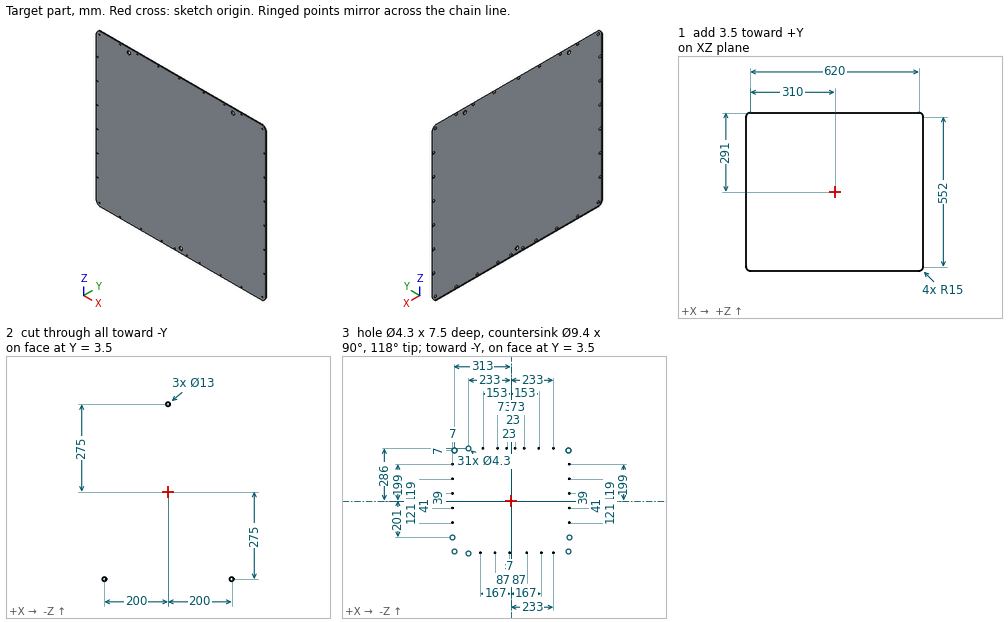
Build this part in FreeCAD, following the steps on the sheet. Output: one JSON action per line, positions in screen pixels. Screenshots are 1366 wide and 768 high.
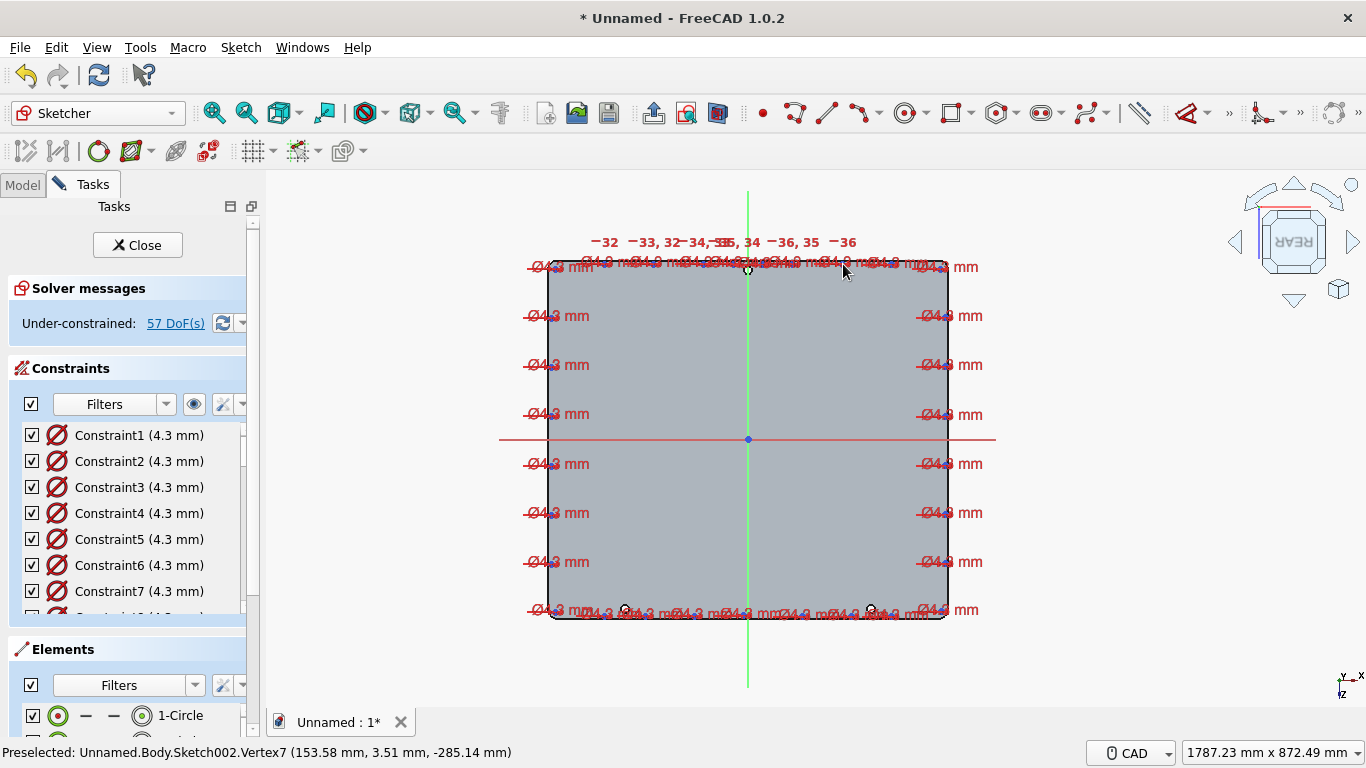
{"action": "left_click", "coordinate": [552, 318]}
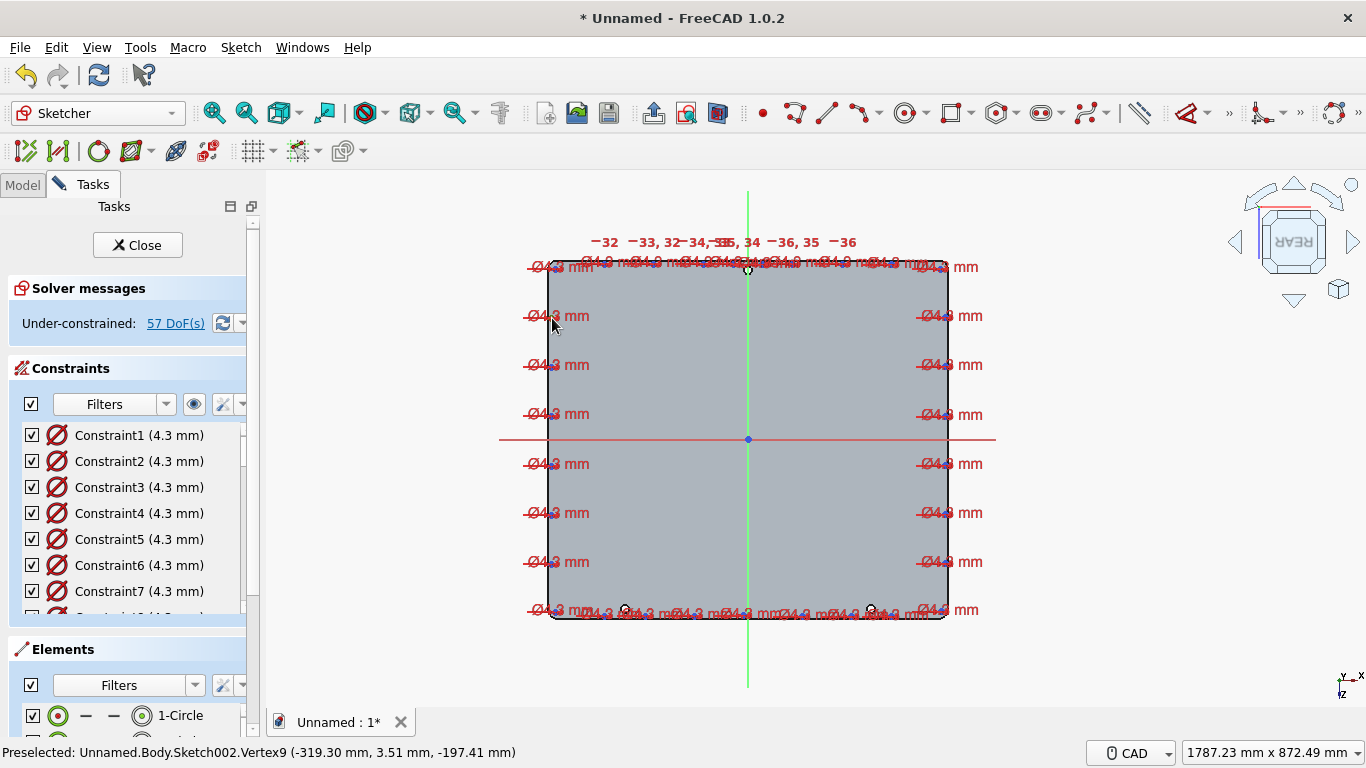
{"action": "left_click", "coordinate": [552, 367]}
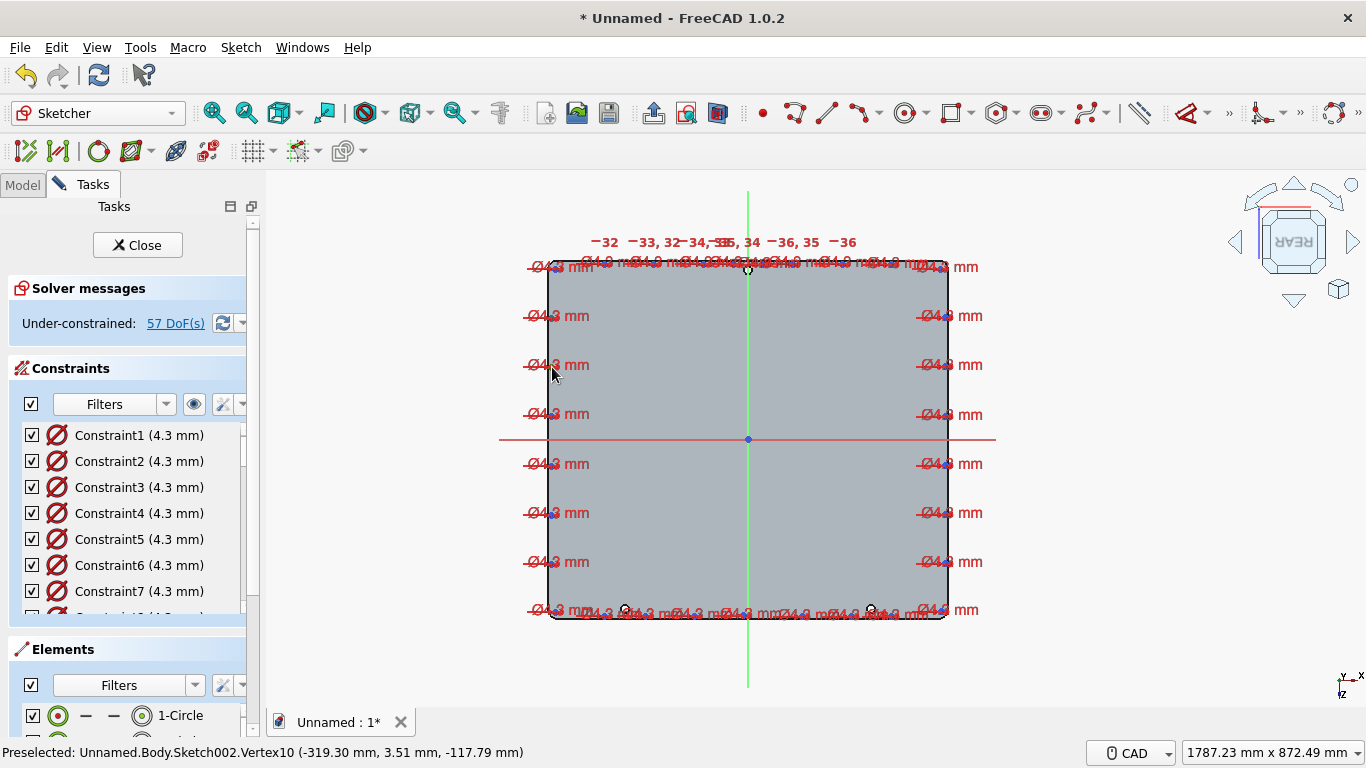
{"action": "key", "text": "v"}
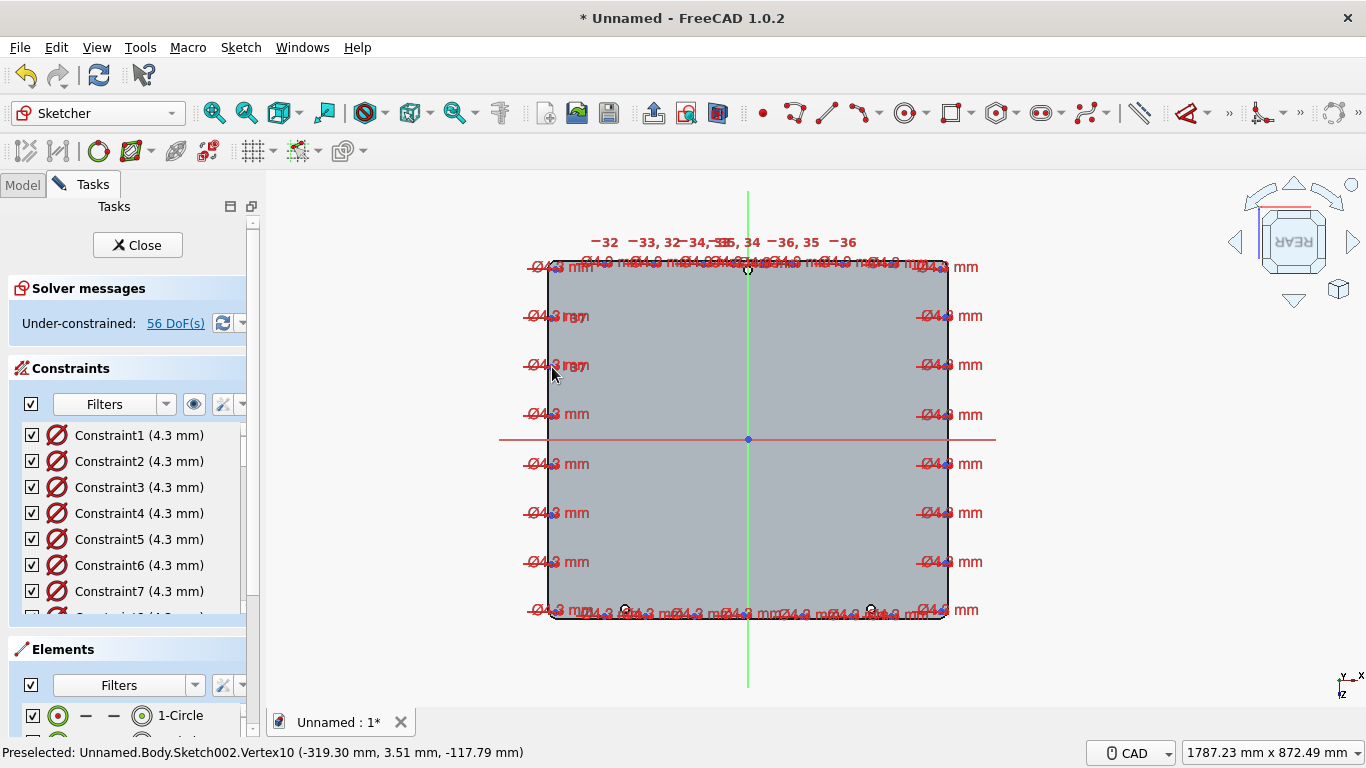
{"action": "left_click", "coordinate": [552, 367]}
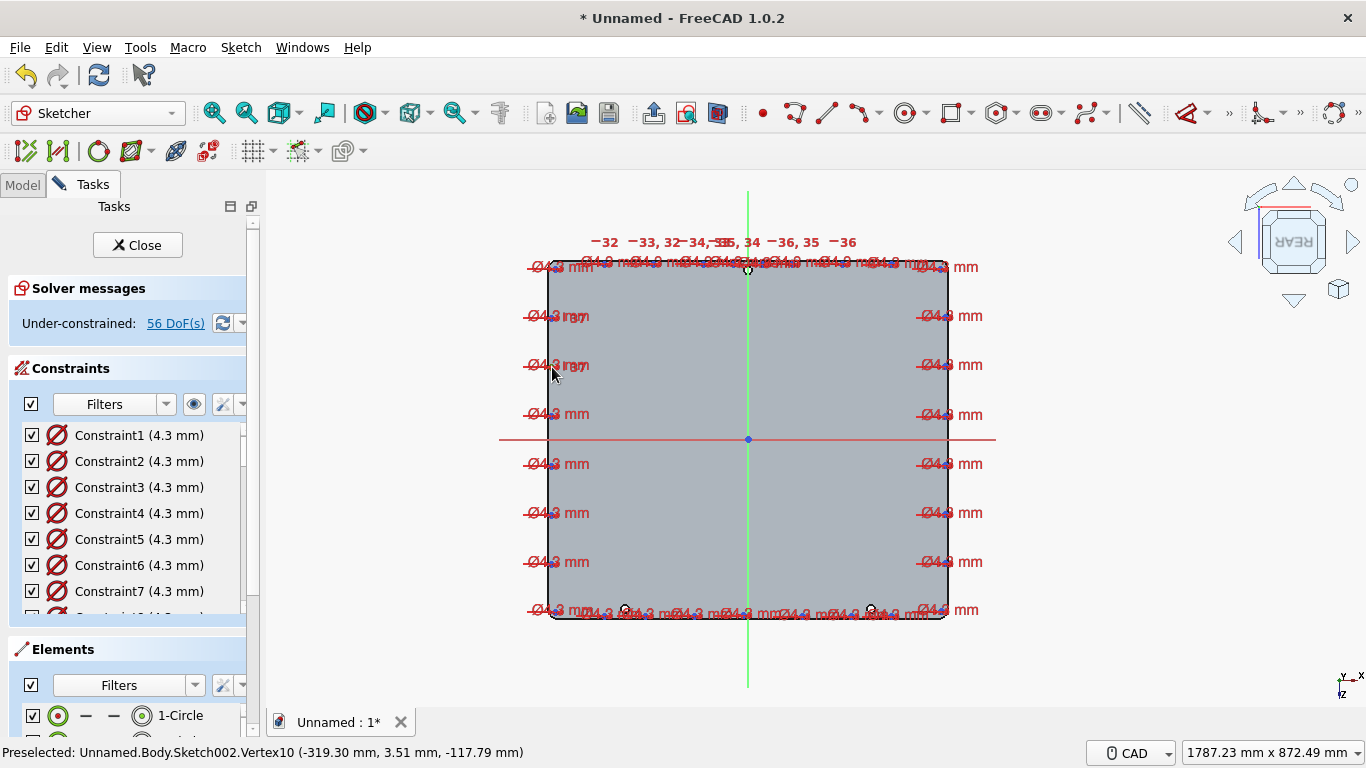
{"action": "left_click", "coordinate": [552, 416]}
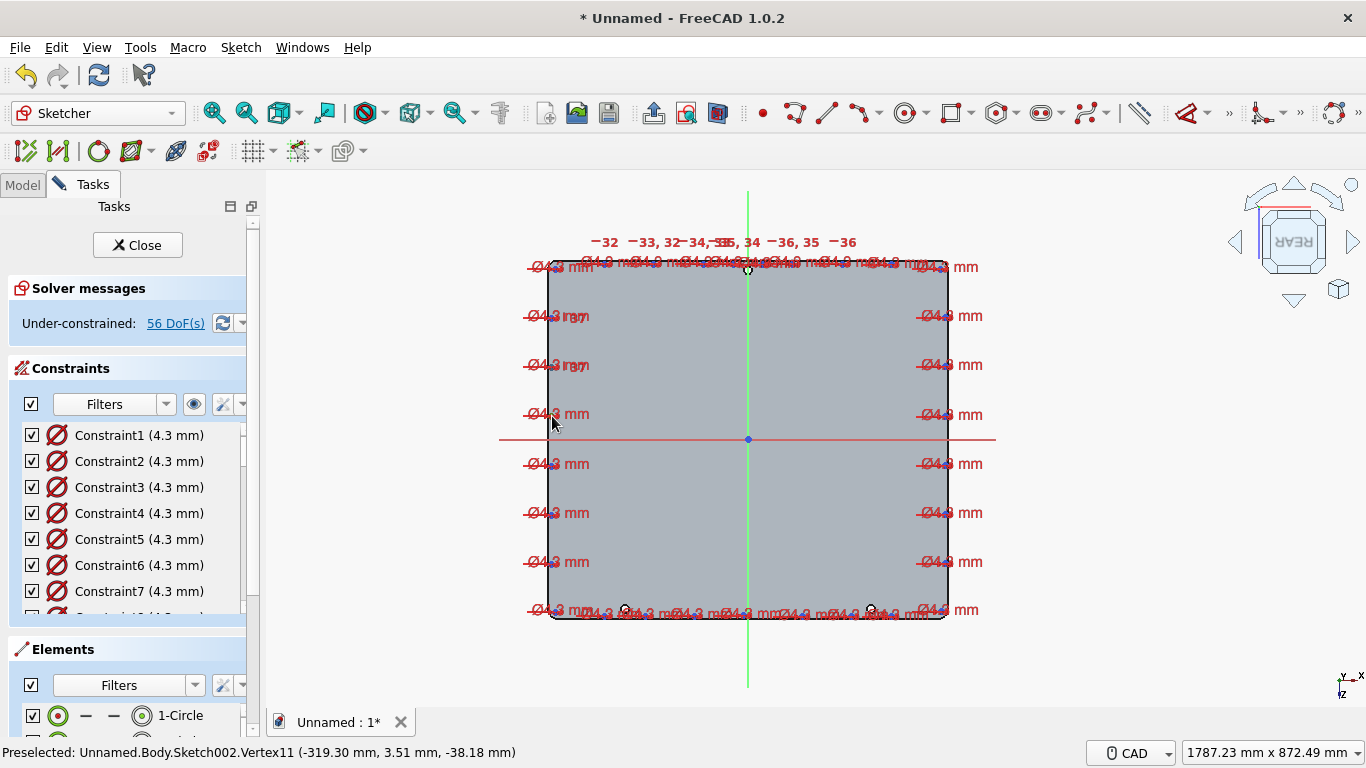
{"action": "key", "text": "v"}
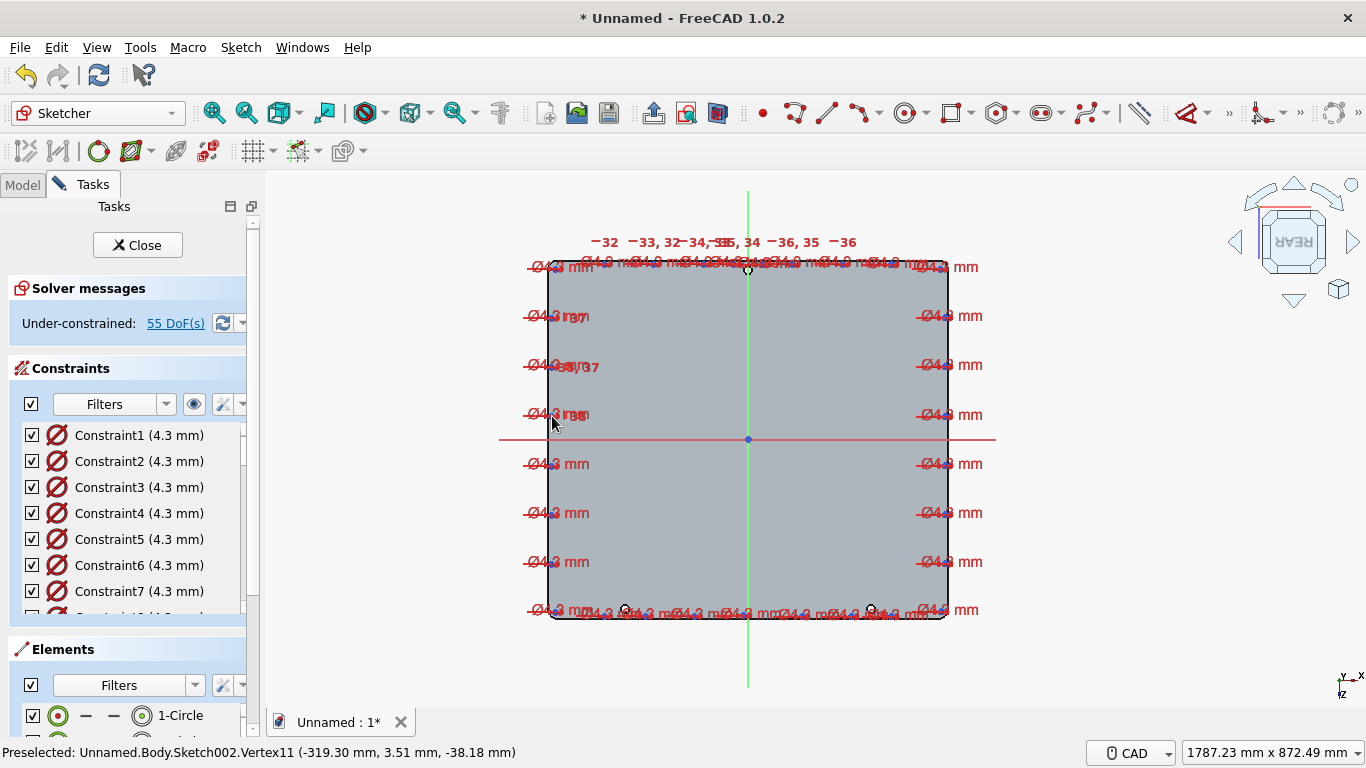
{"action": "left_click", "coordinate": [552, 416]}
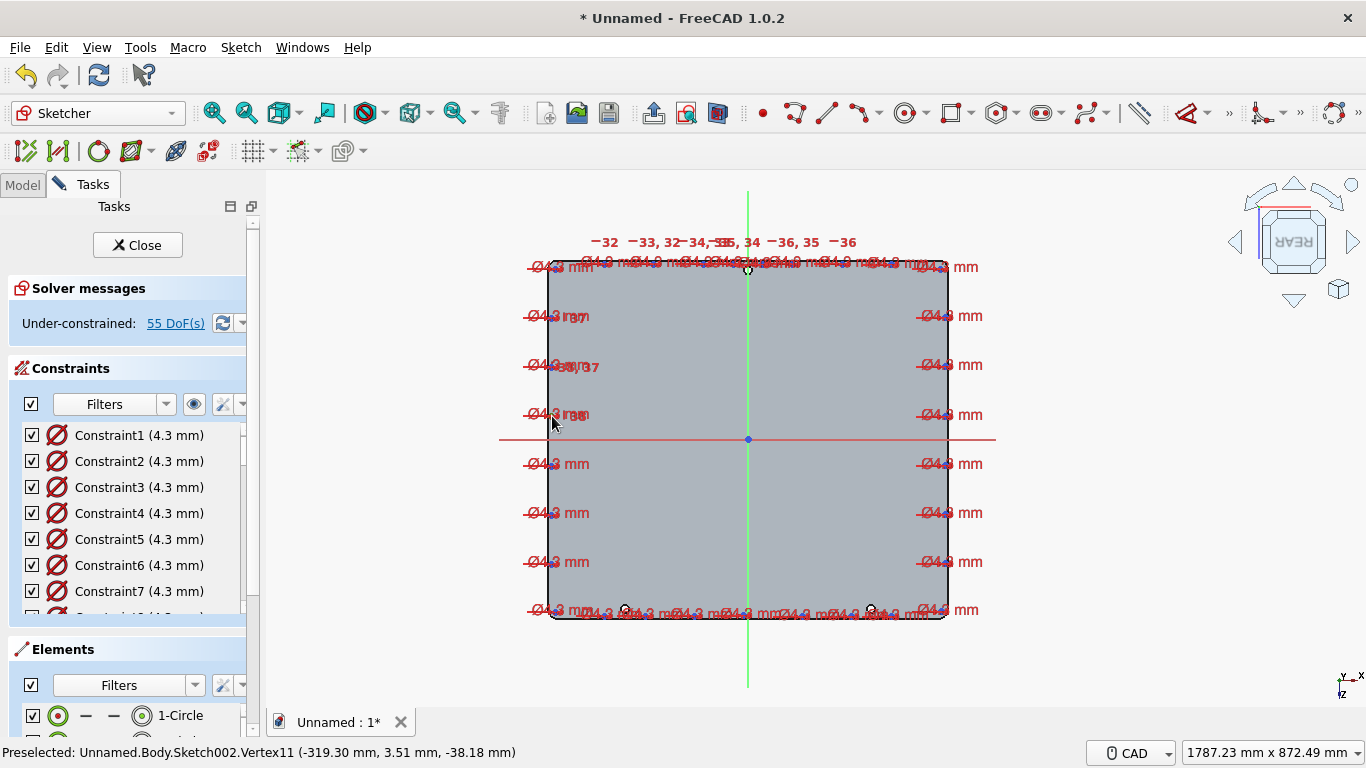
{"action": "left_click", "coordinate": [552, 466]}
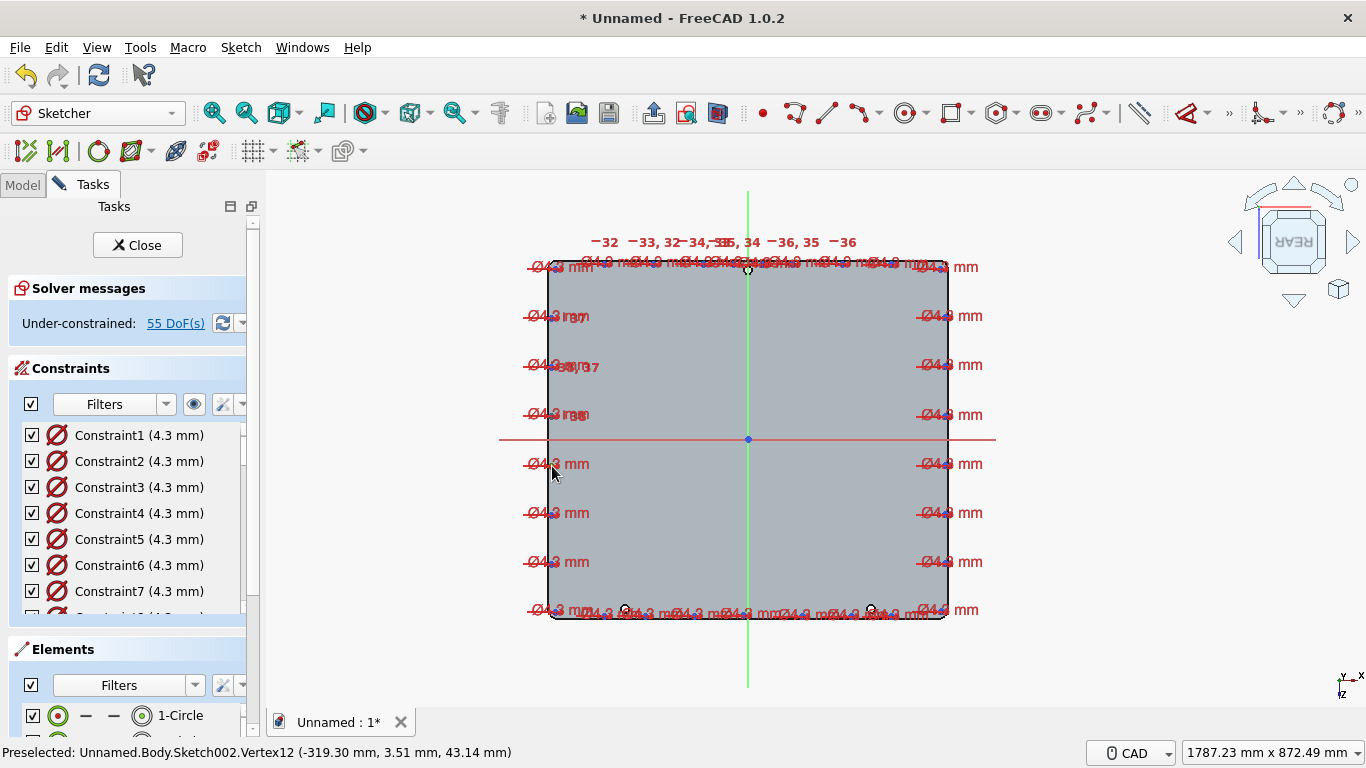
{"action": "key", "text": "v"}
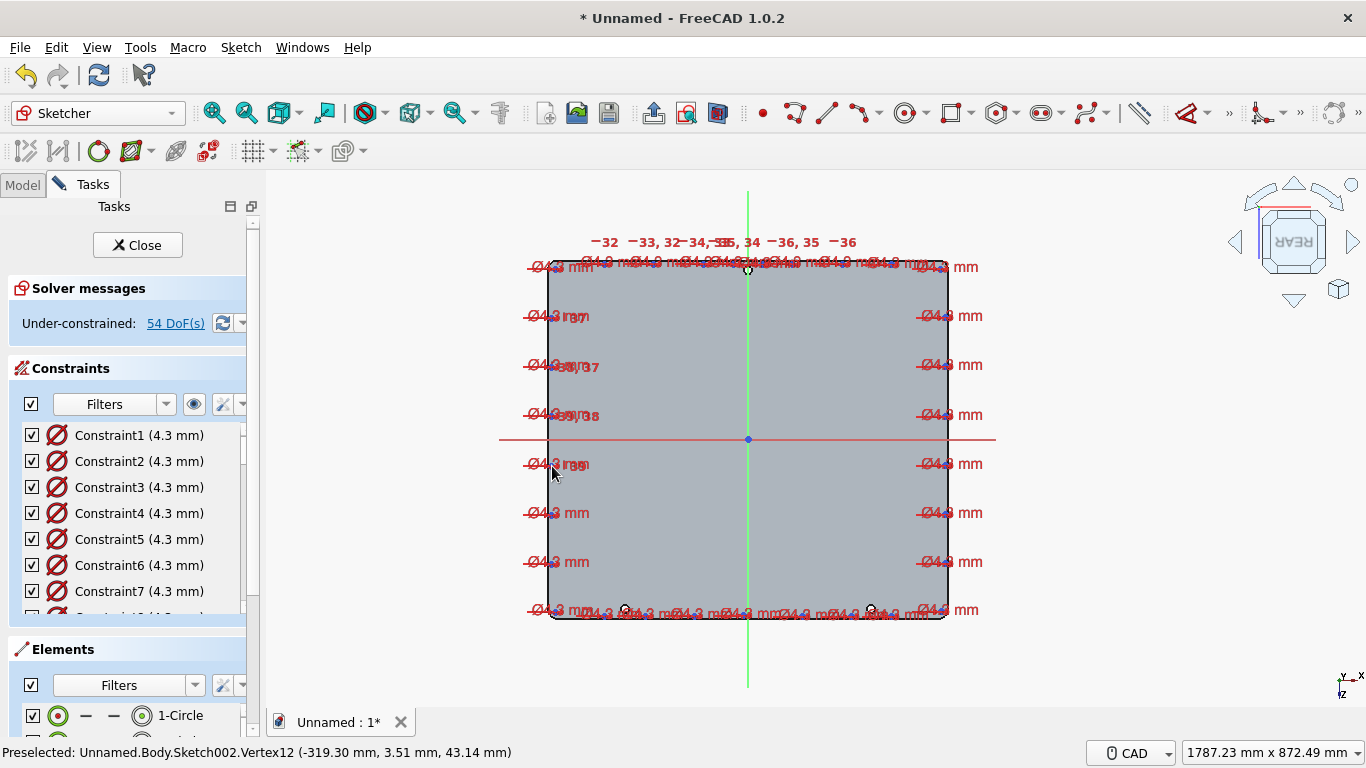
{"action": "left_click", "coordinate": [552, 466]}